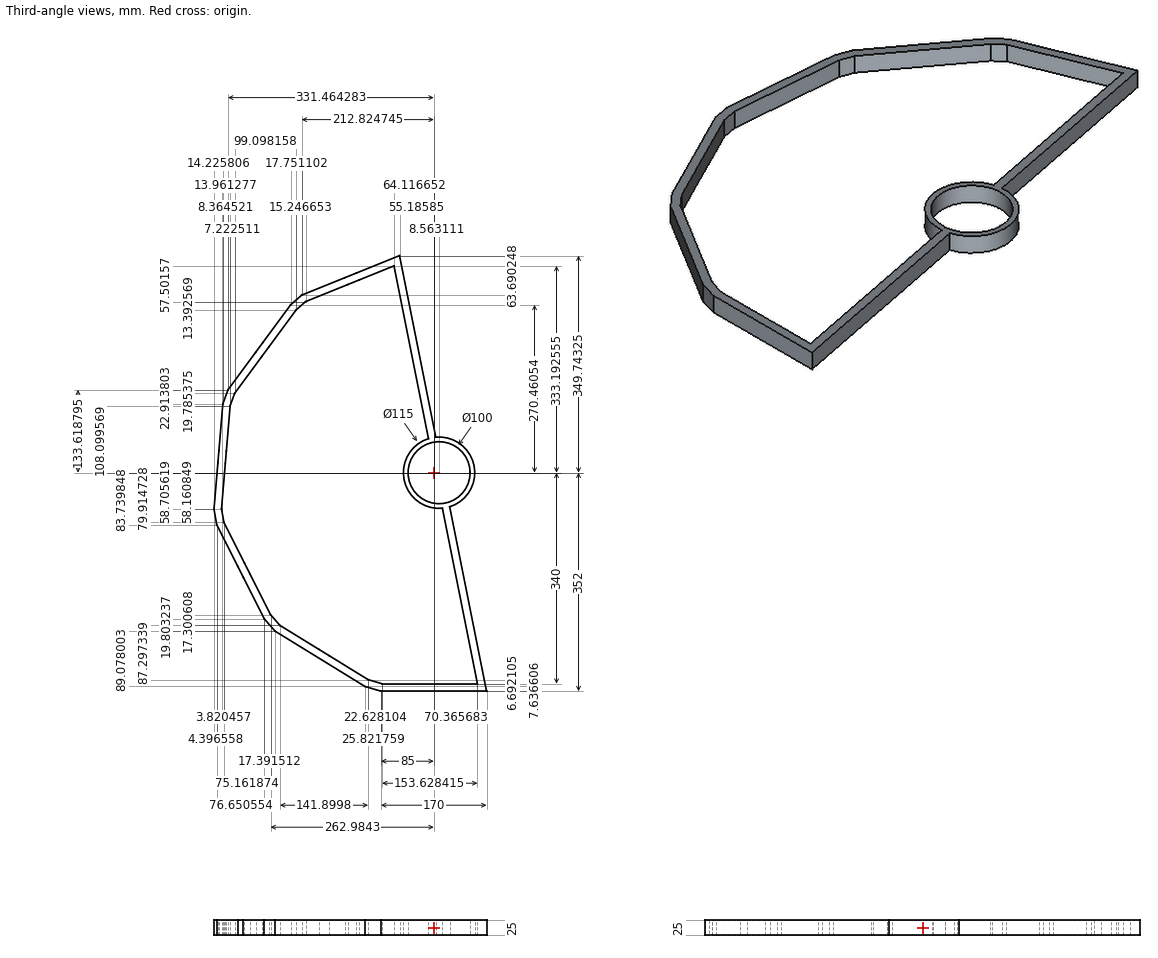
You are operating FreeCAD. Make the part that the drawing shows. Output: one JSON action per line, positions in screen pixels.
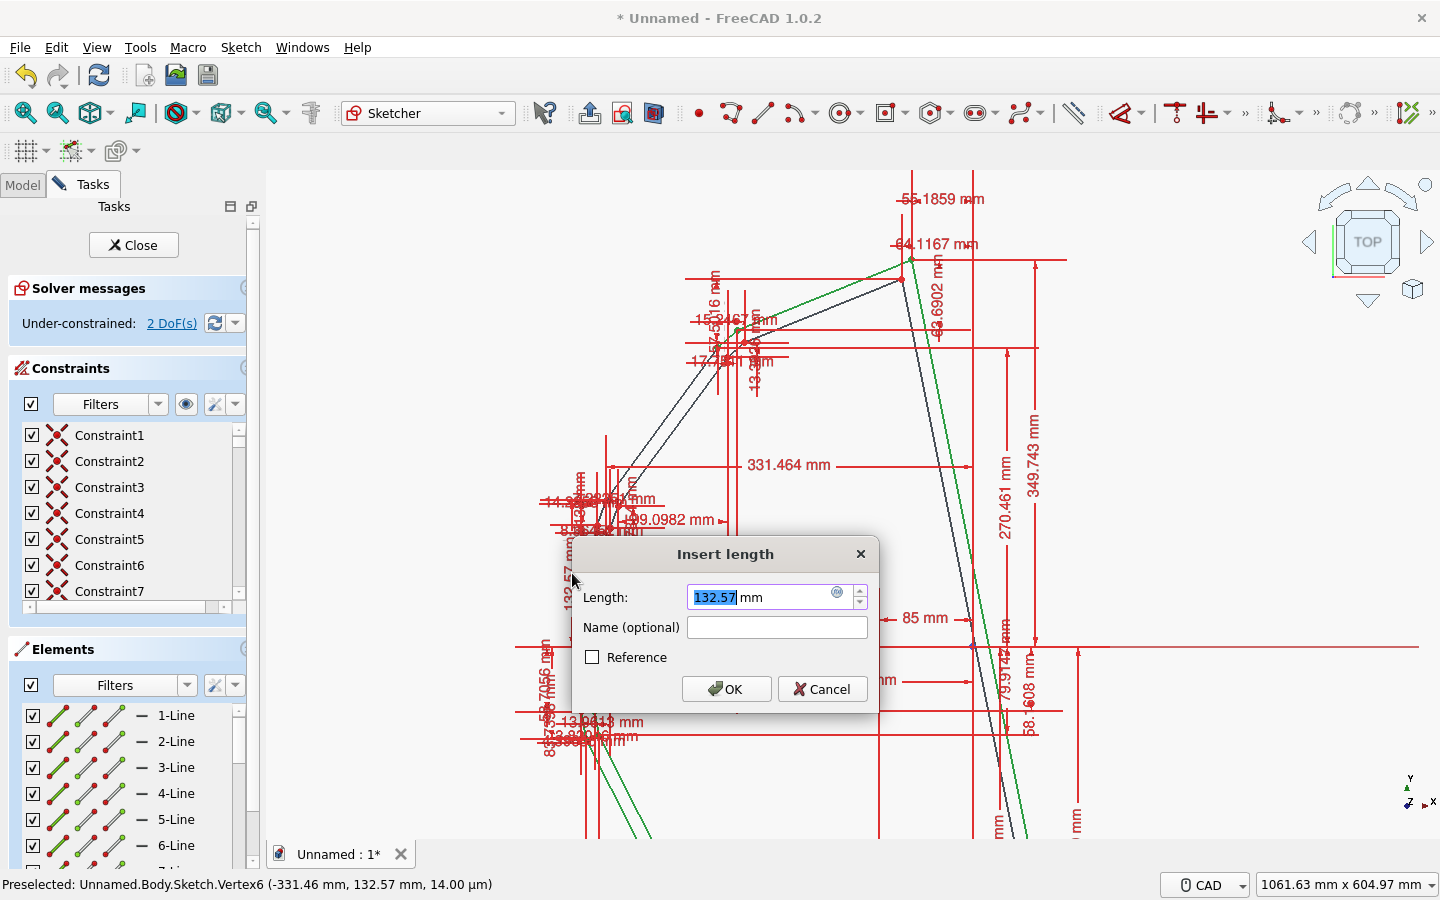
{"action": "type", "text": "133.618795"}
{"action": "key", "text": "Return"}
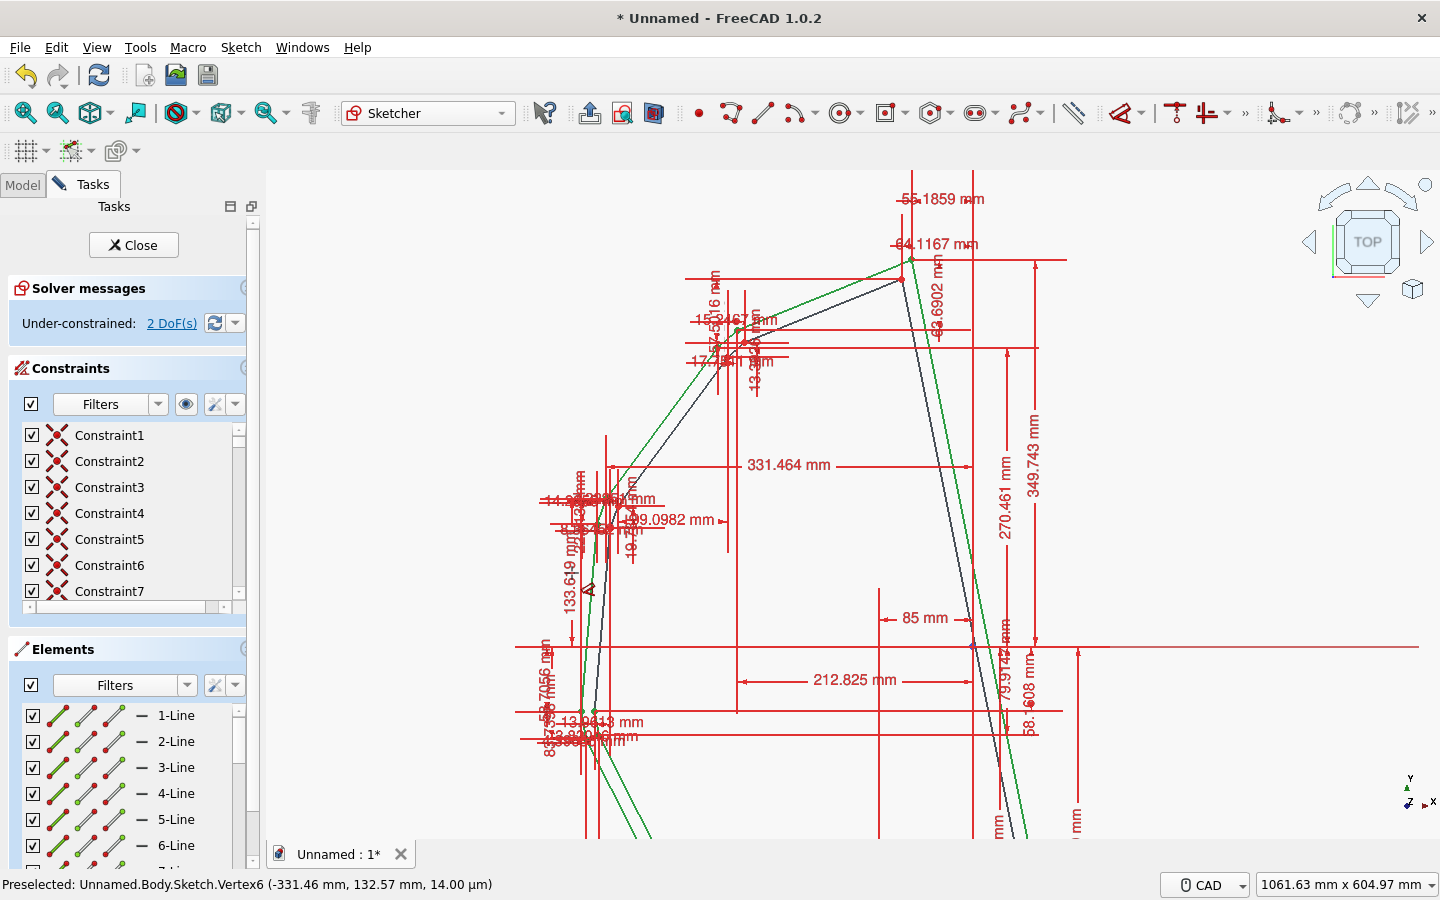
{"action": "left_click", "coordinate": [902, 279]}
{"action": "left_click", "coordinate": [1007, 378]}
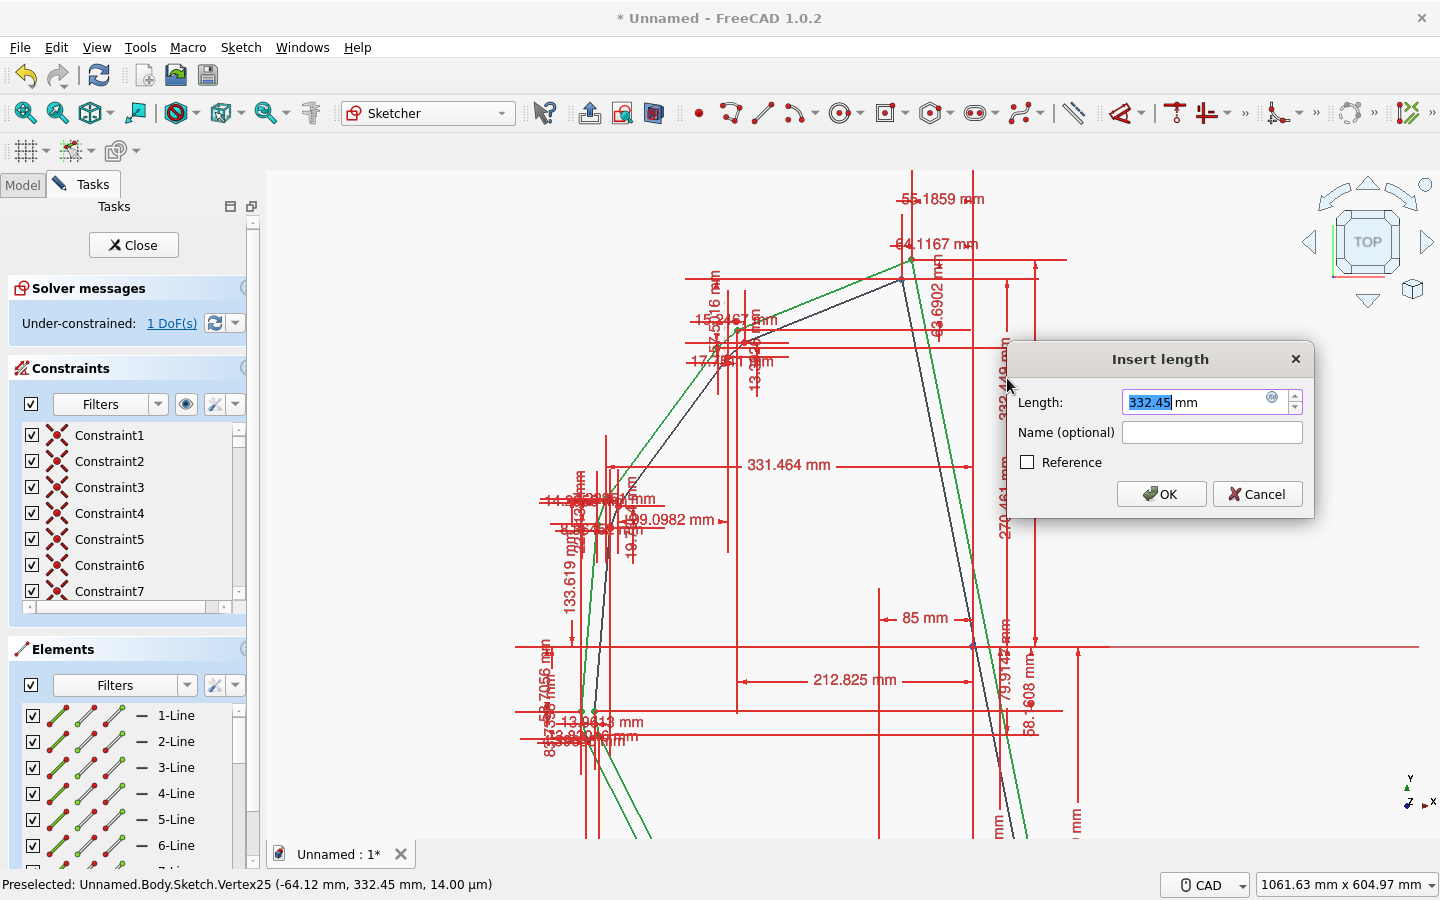
{"action": "type", "text": "333.192555"}
{"action": "key", "text": "Return"}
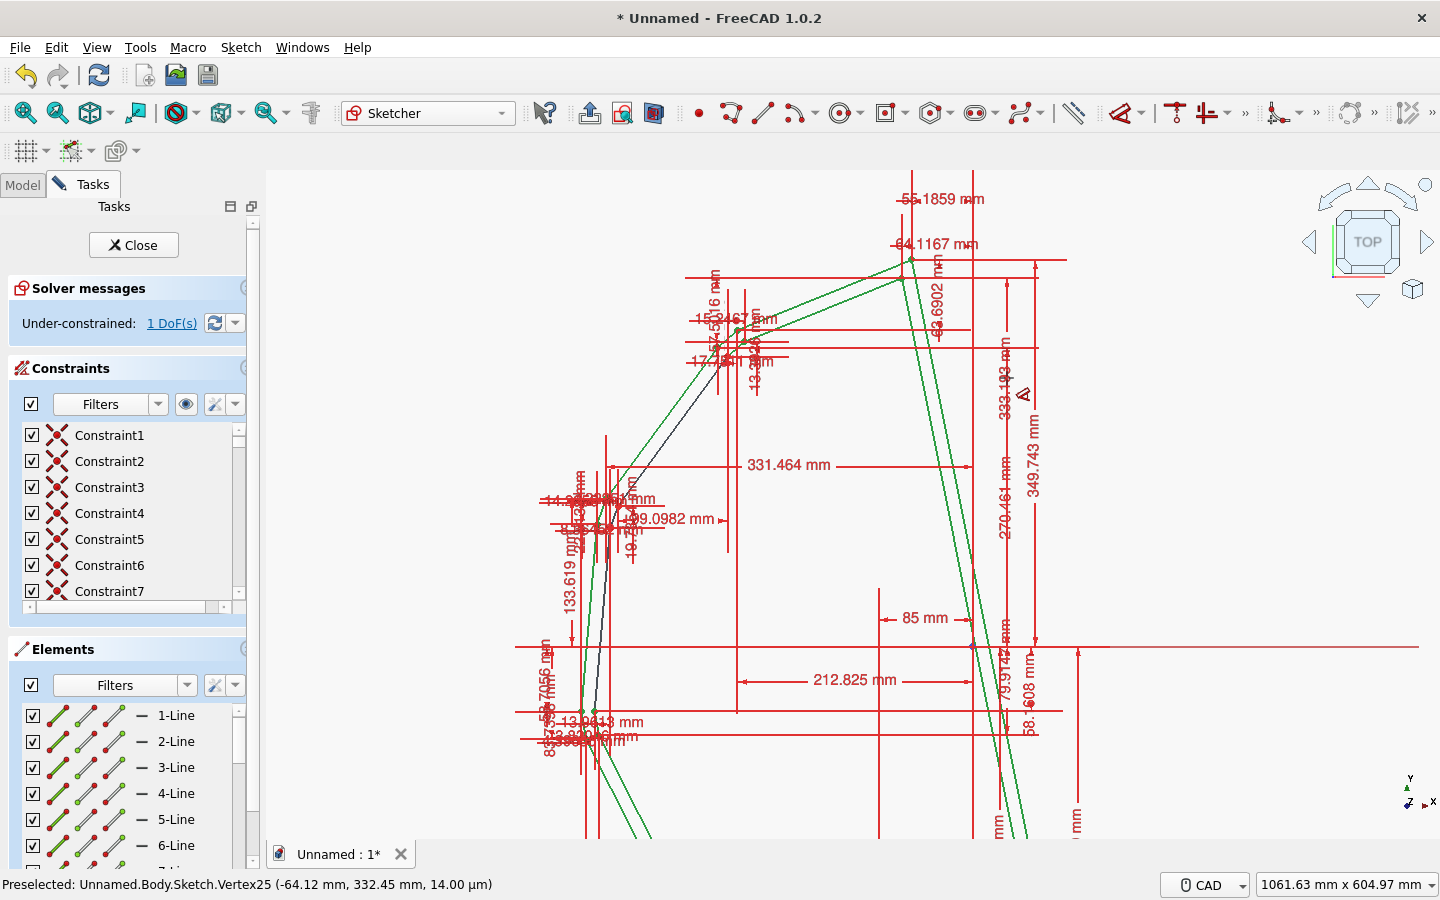
{"action": "left_click", "coordinate": [610, 528]}
{"action": "left_click", "coordinate": [576, 615]}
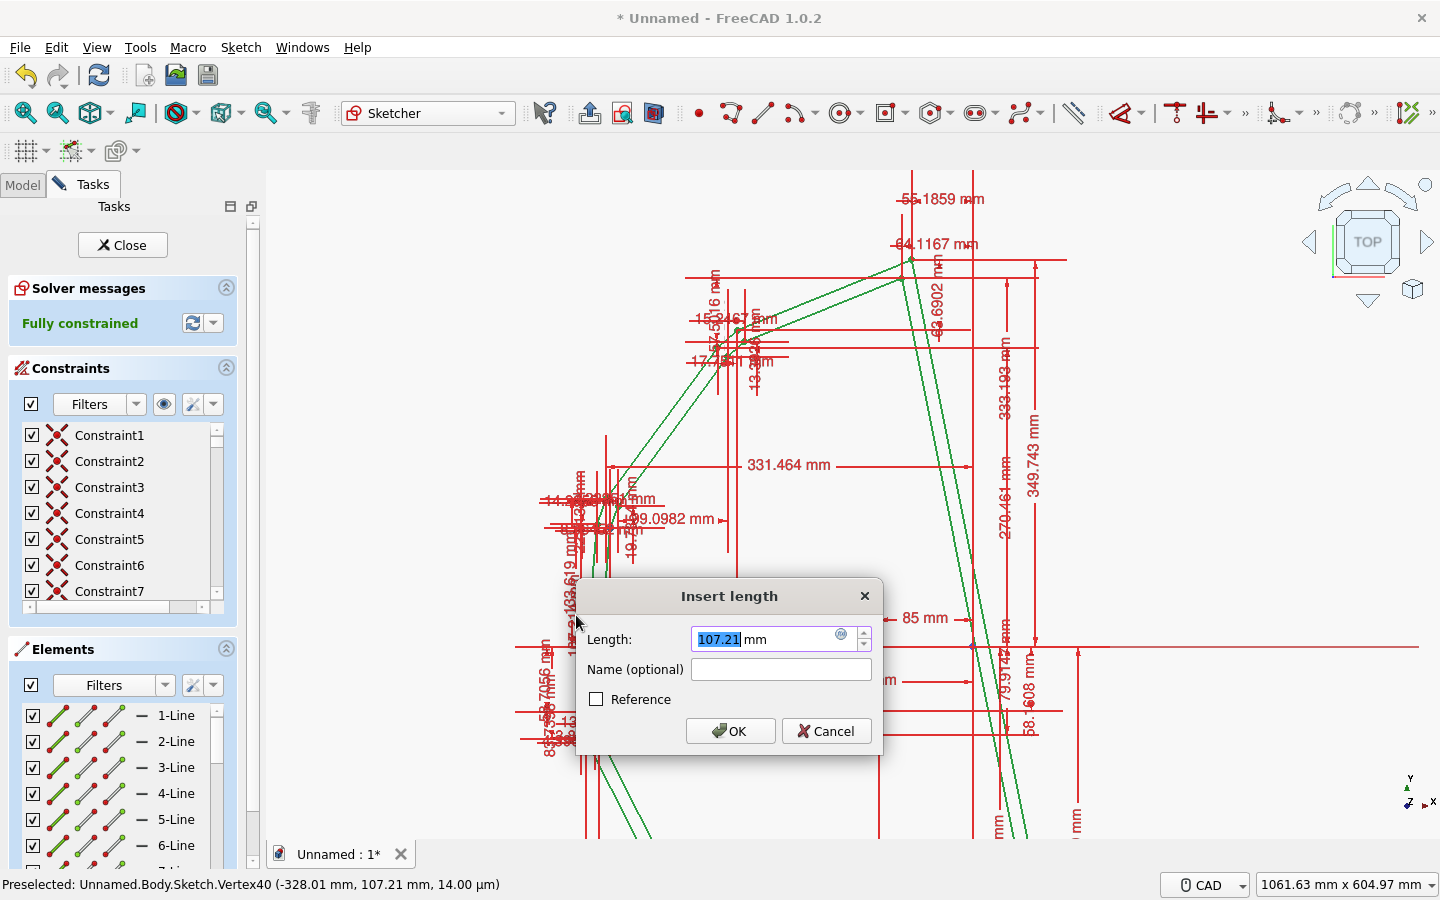
{"action": "type", "text": "108.099569"}
{"action": "key", "text": "Return"}
{"action": "key", "text": "Escape"}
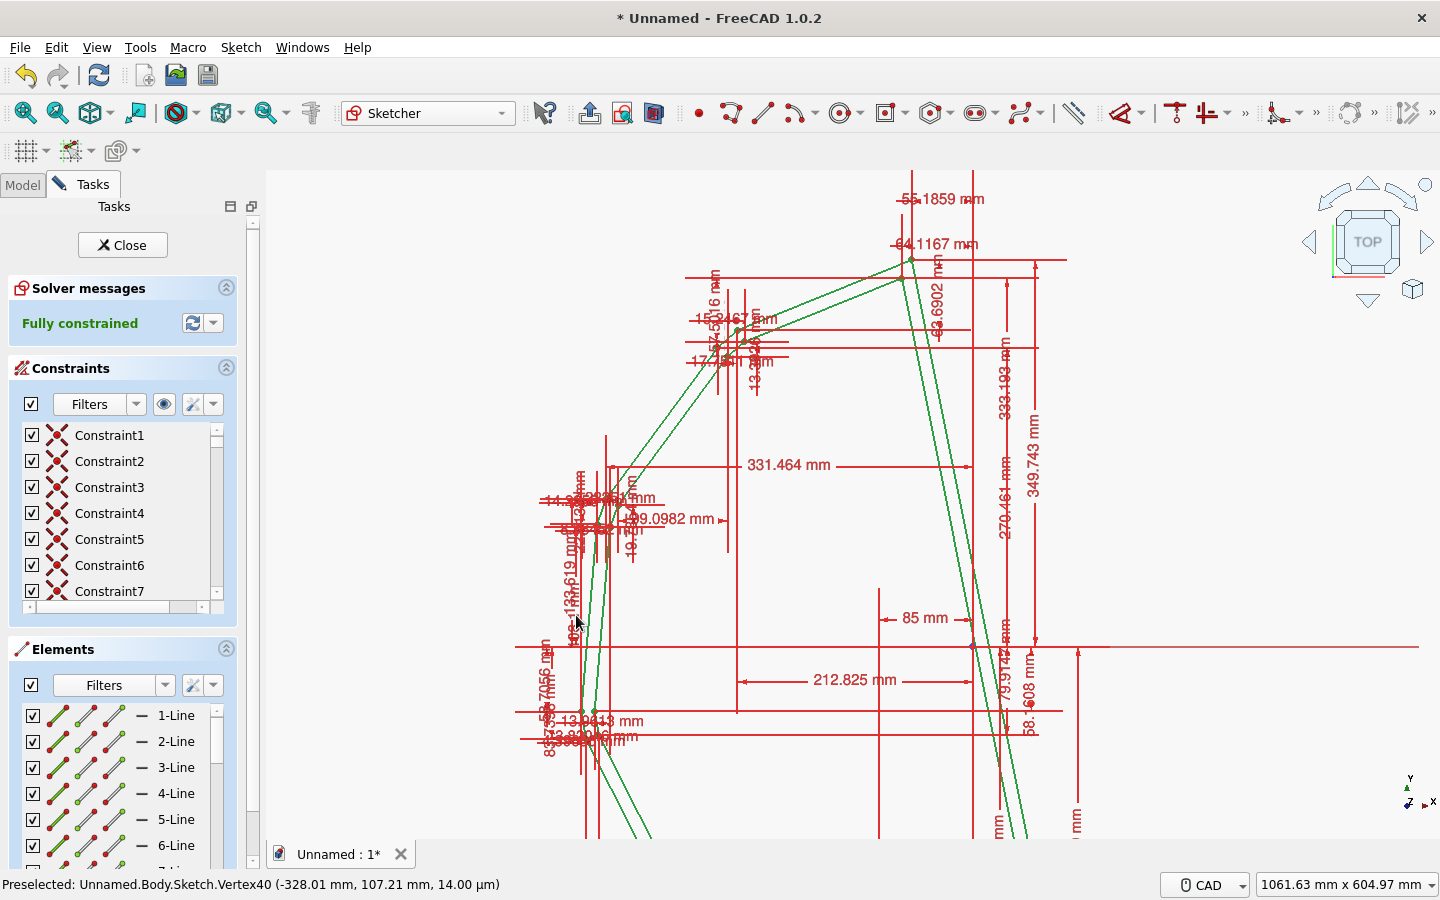
{"action": "left_click", "coordinate": [123, 245]}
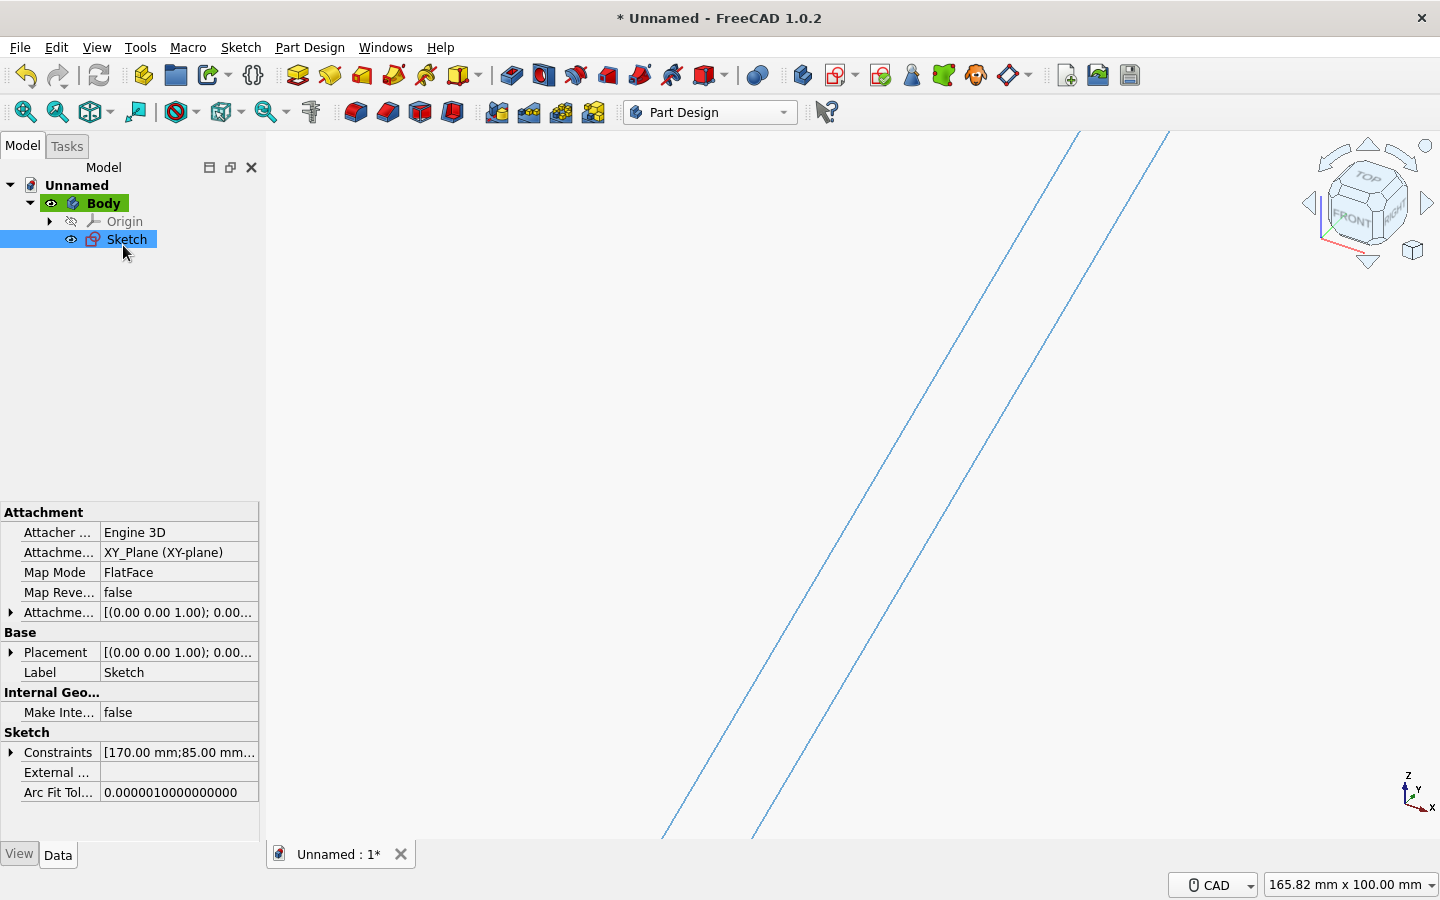
{"action": "left_click", "coordinate": [298, 76]}